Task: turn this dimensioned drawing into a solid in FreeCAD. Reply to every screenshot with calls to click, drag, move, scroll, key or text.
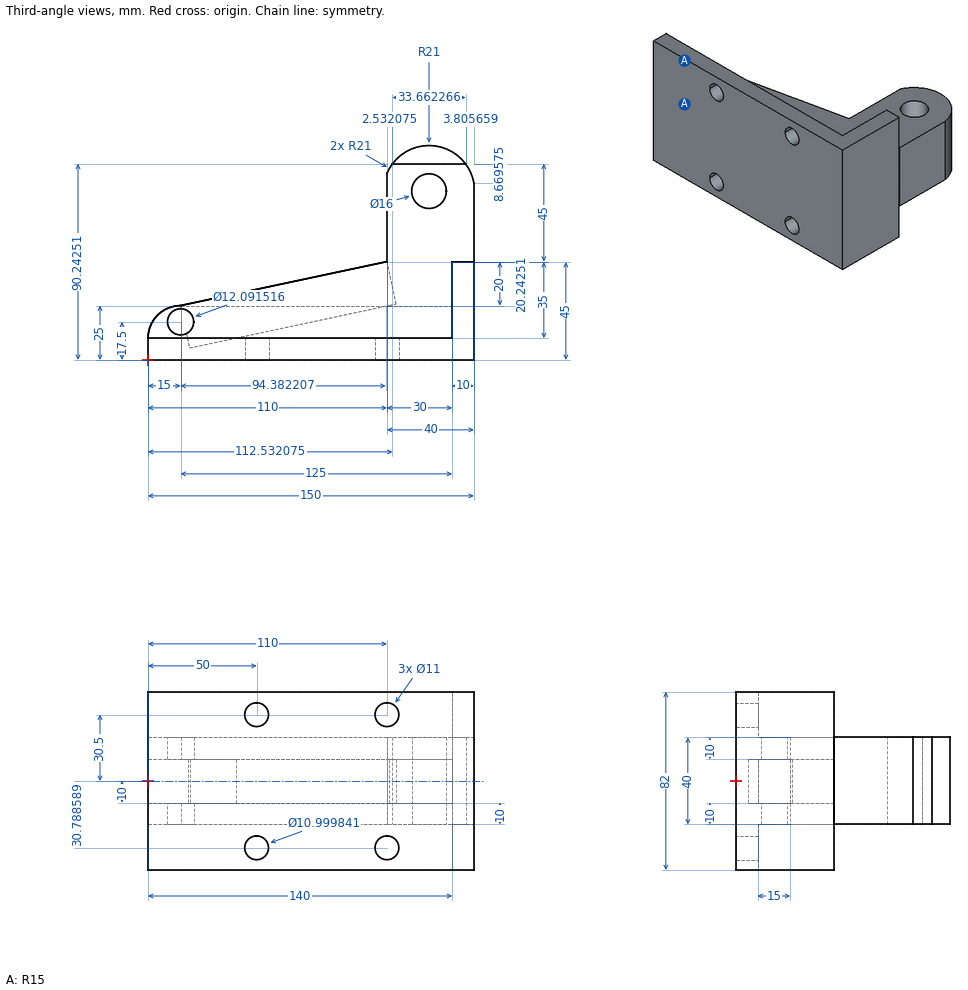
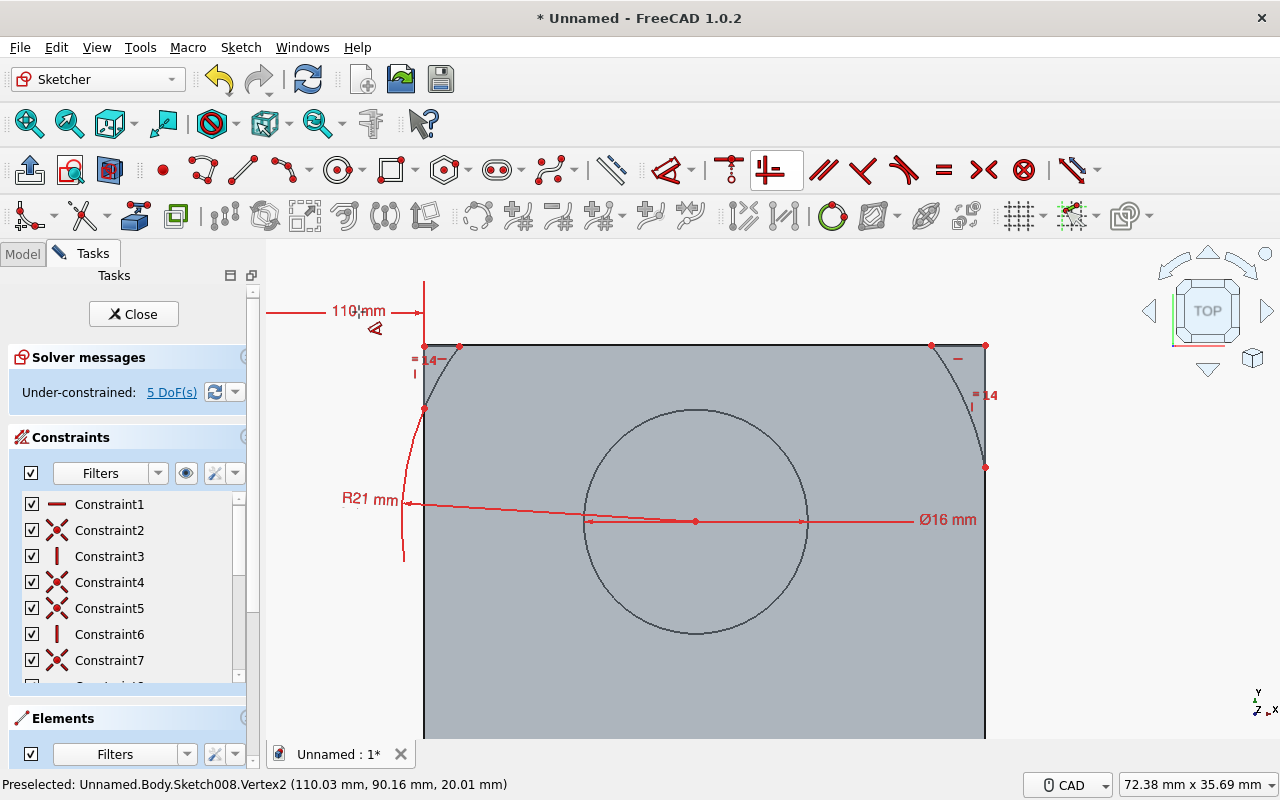
click(985, 468)
click(481, 434)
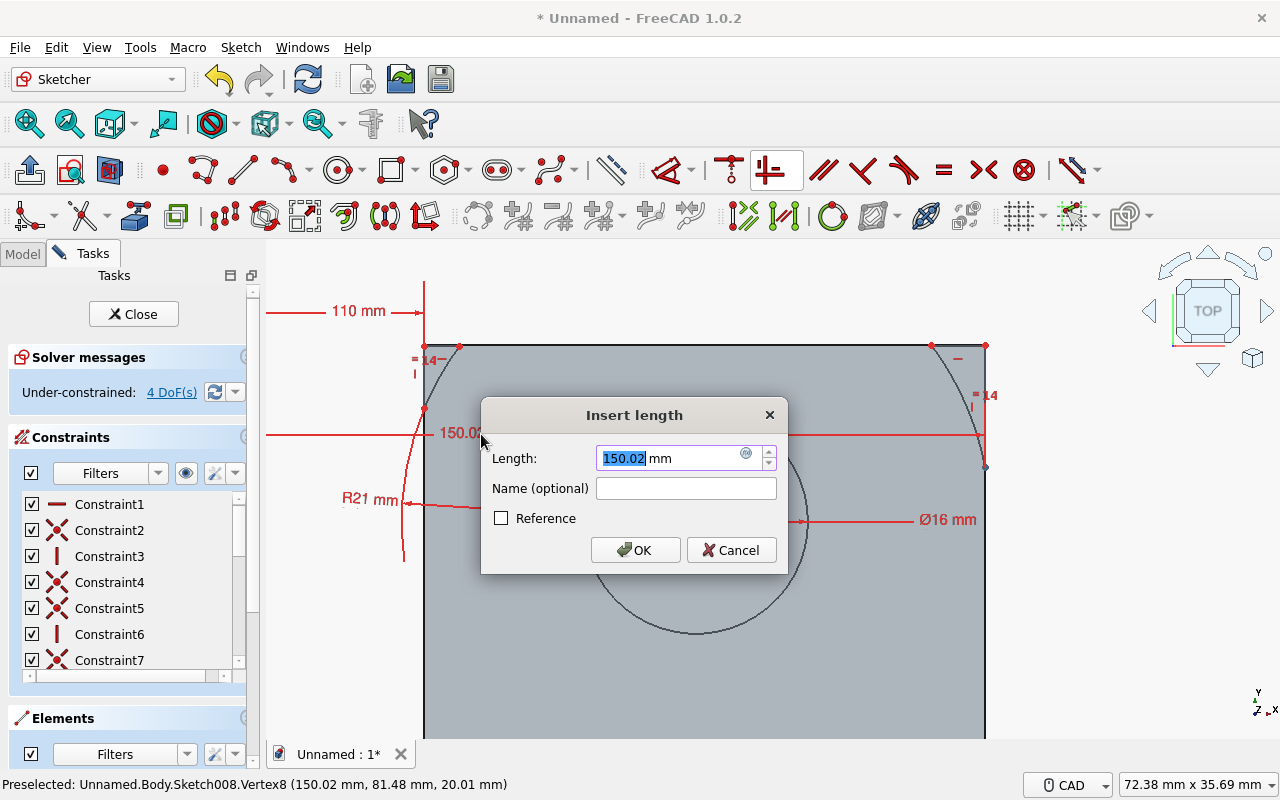
text(150)
key(Return)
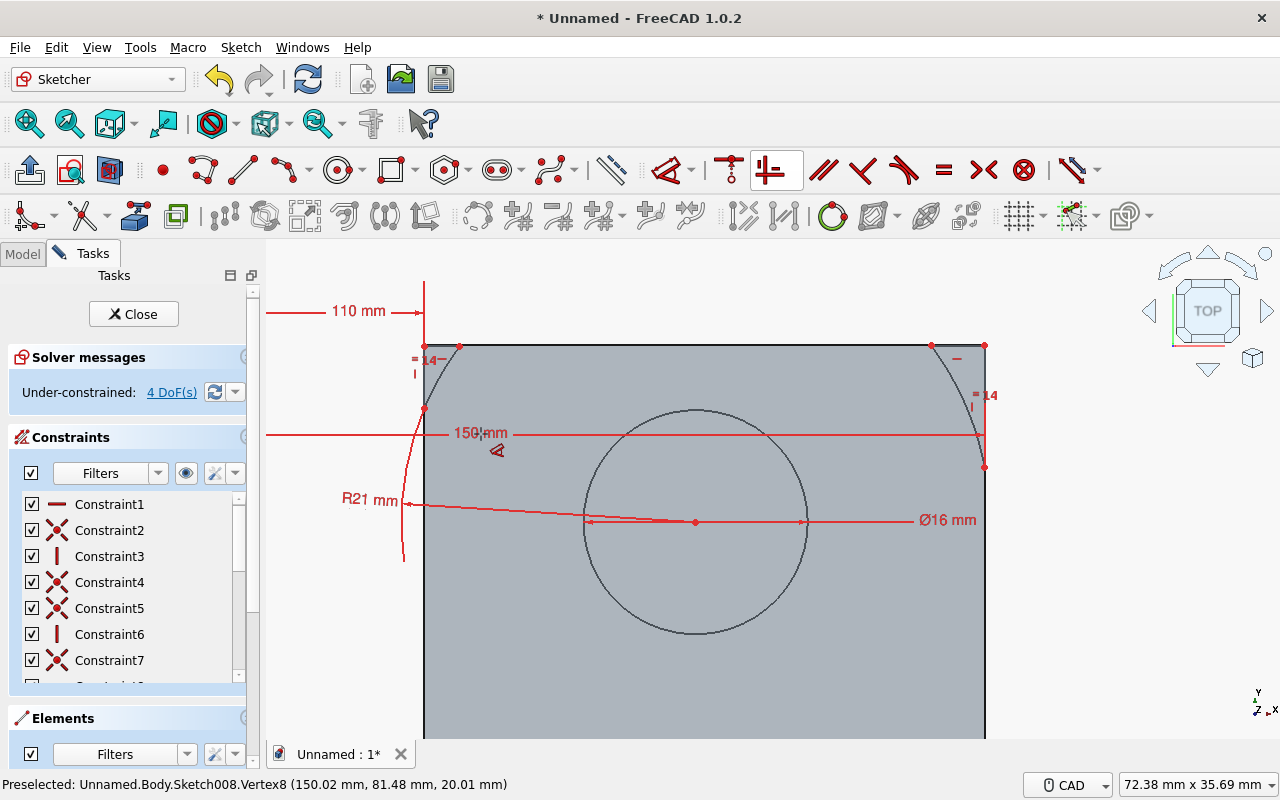
scroll(435, 346, up, 2)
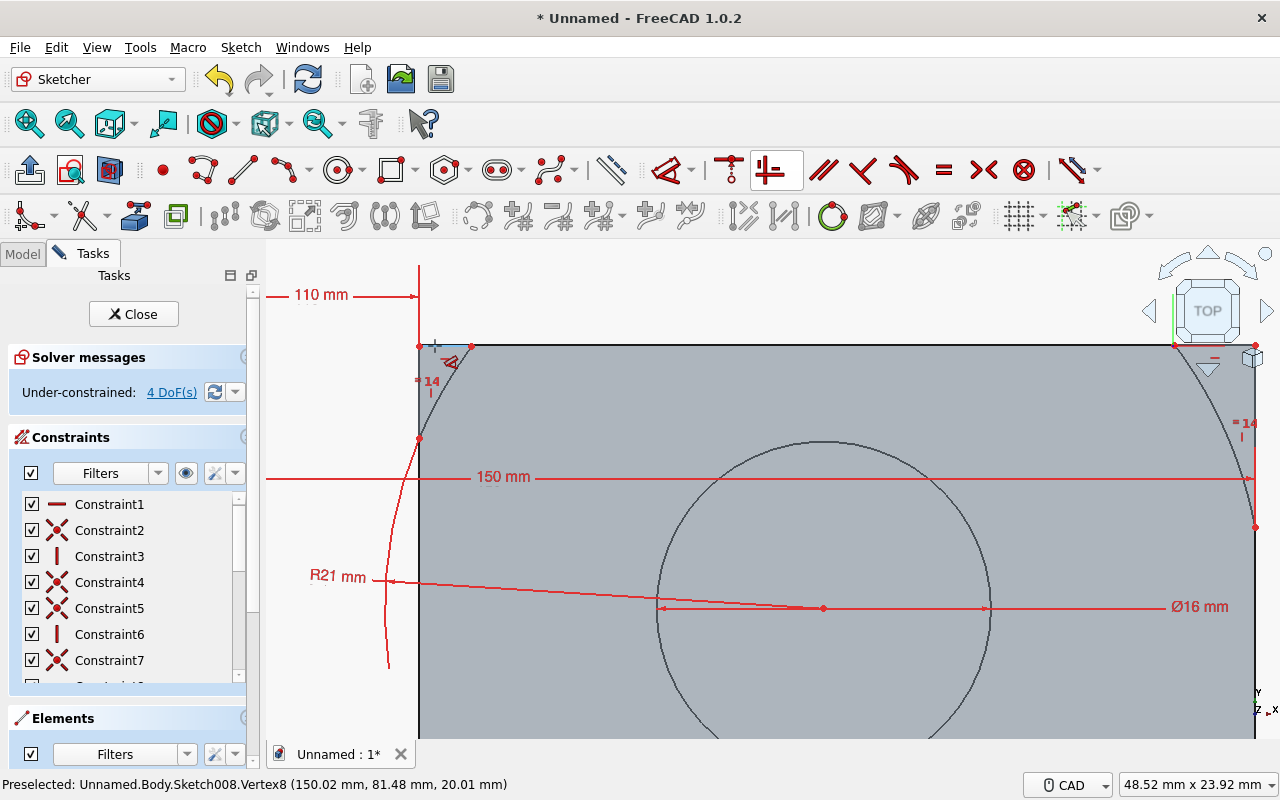
click(435, 346)
click(446, 312)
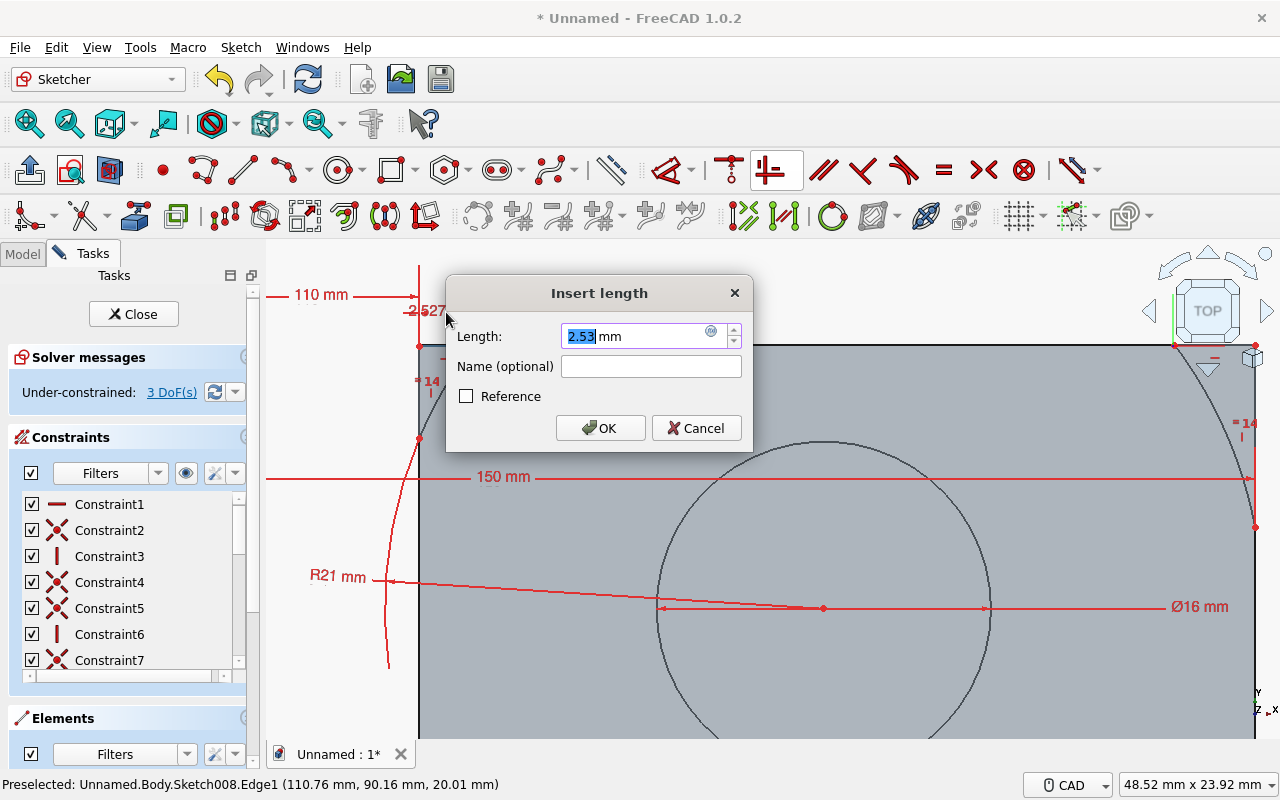
text(2.532075)
key(Return)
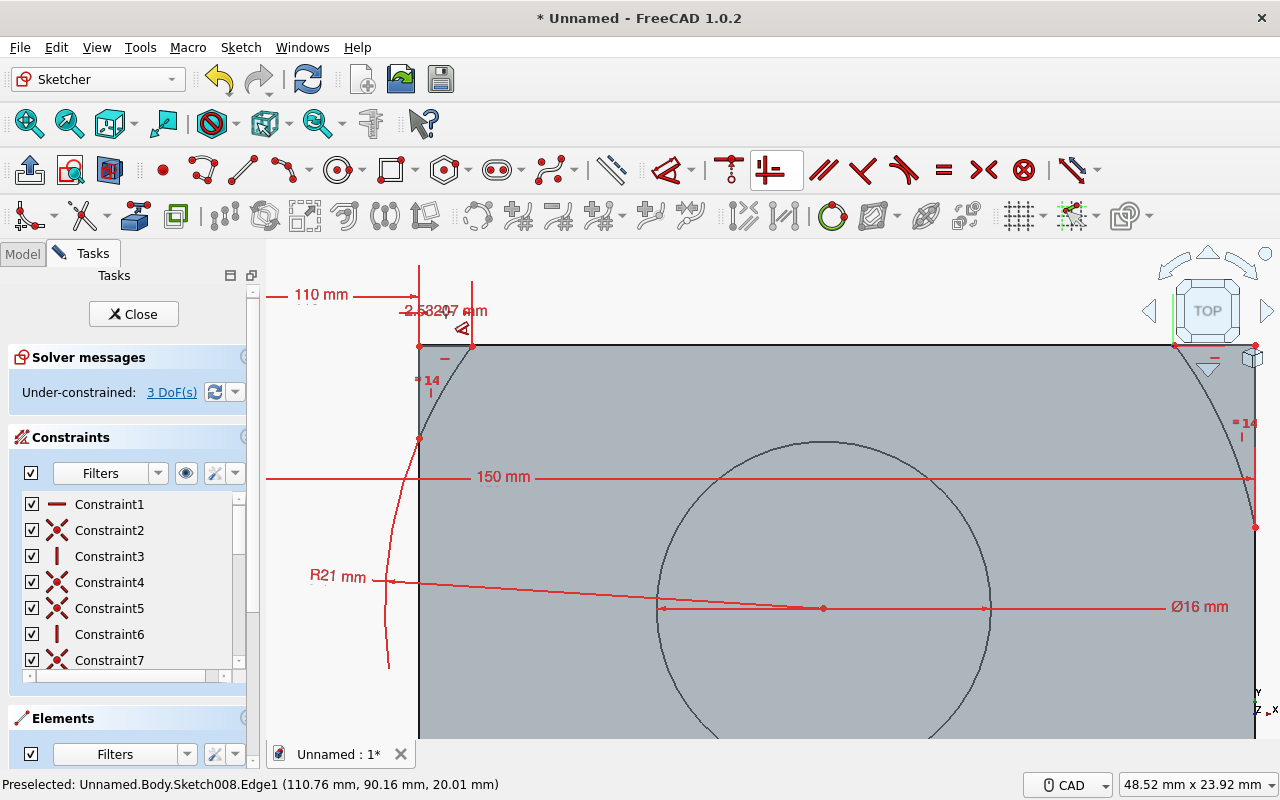
scroll(435, 346, down, 2)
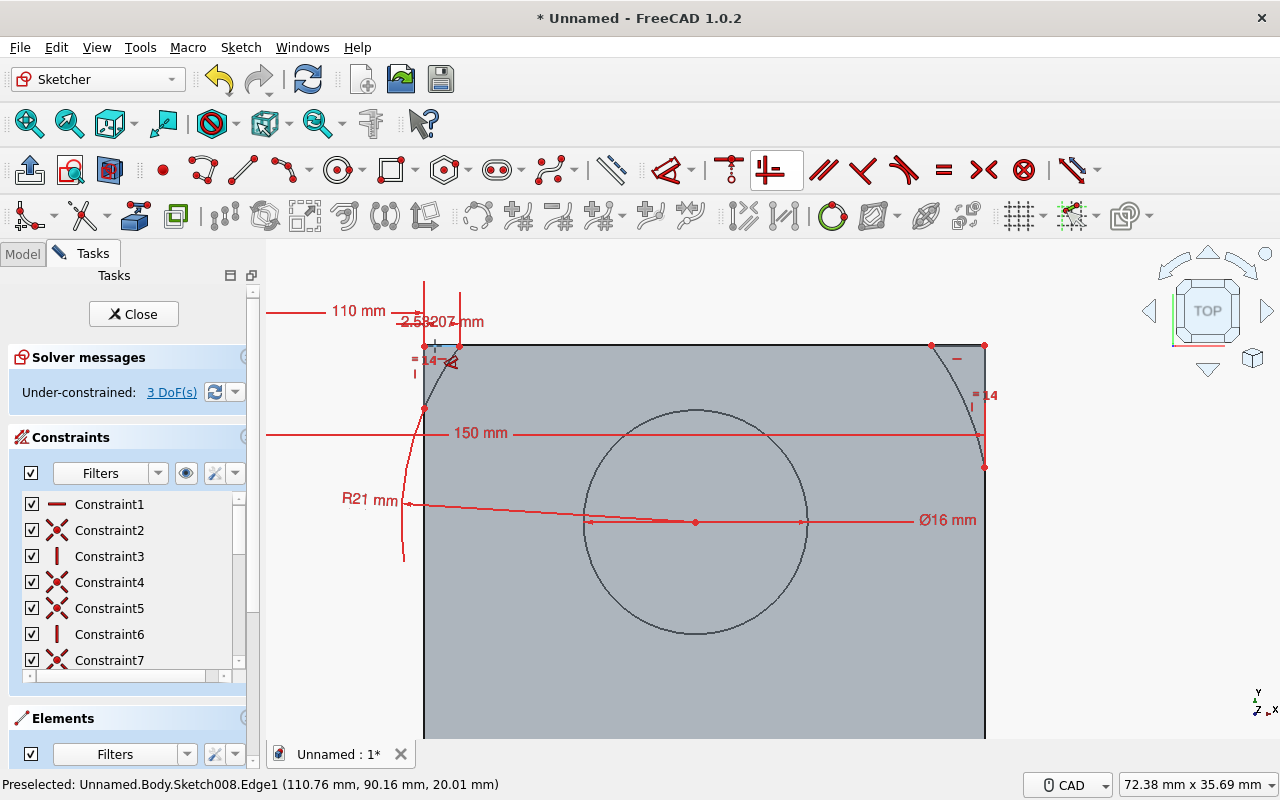
scroll(985, 431, up, 3)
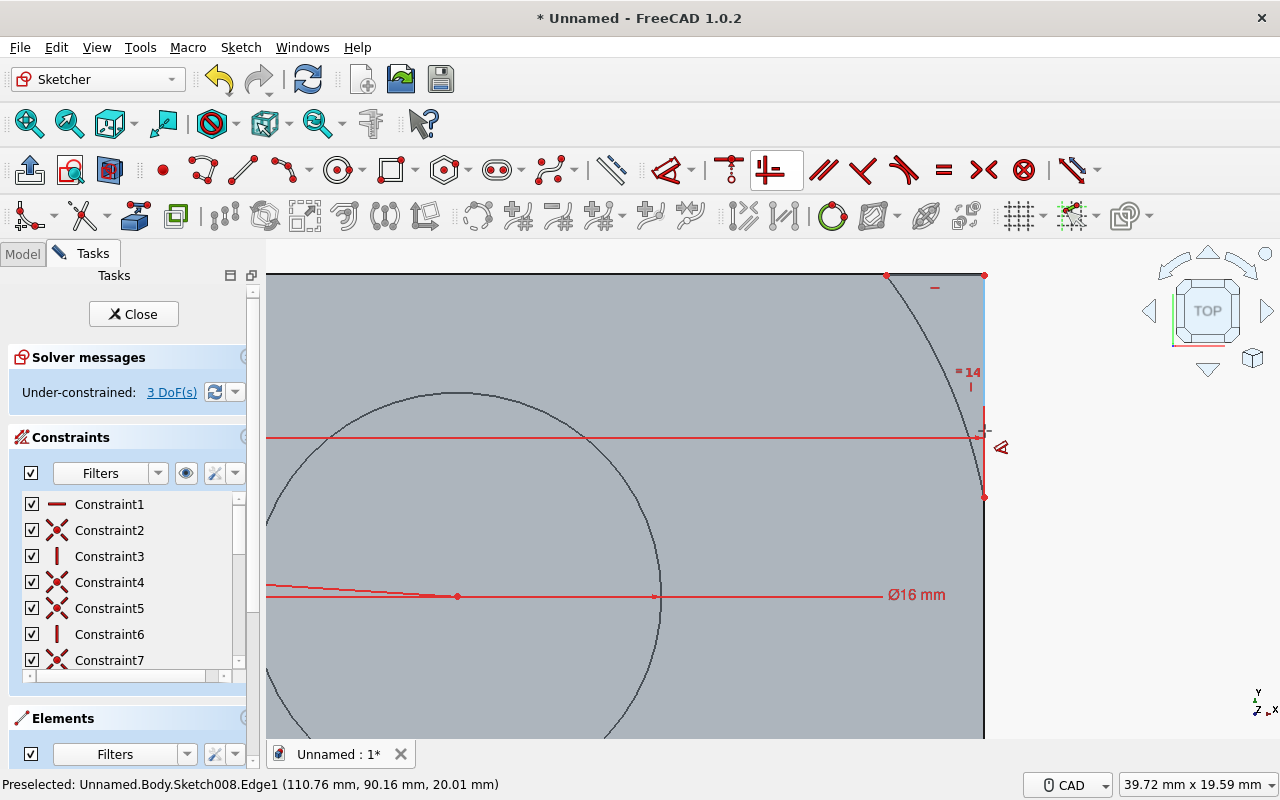
click(984, 431)
click(1018, 387)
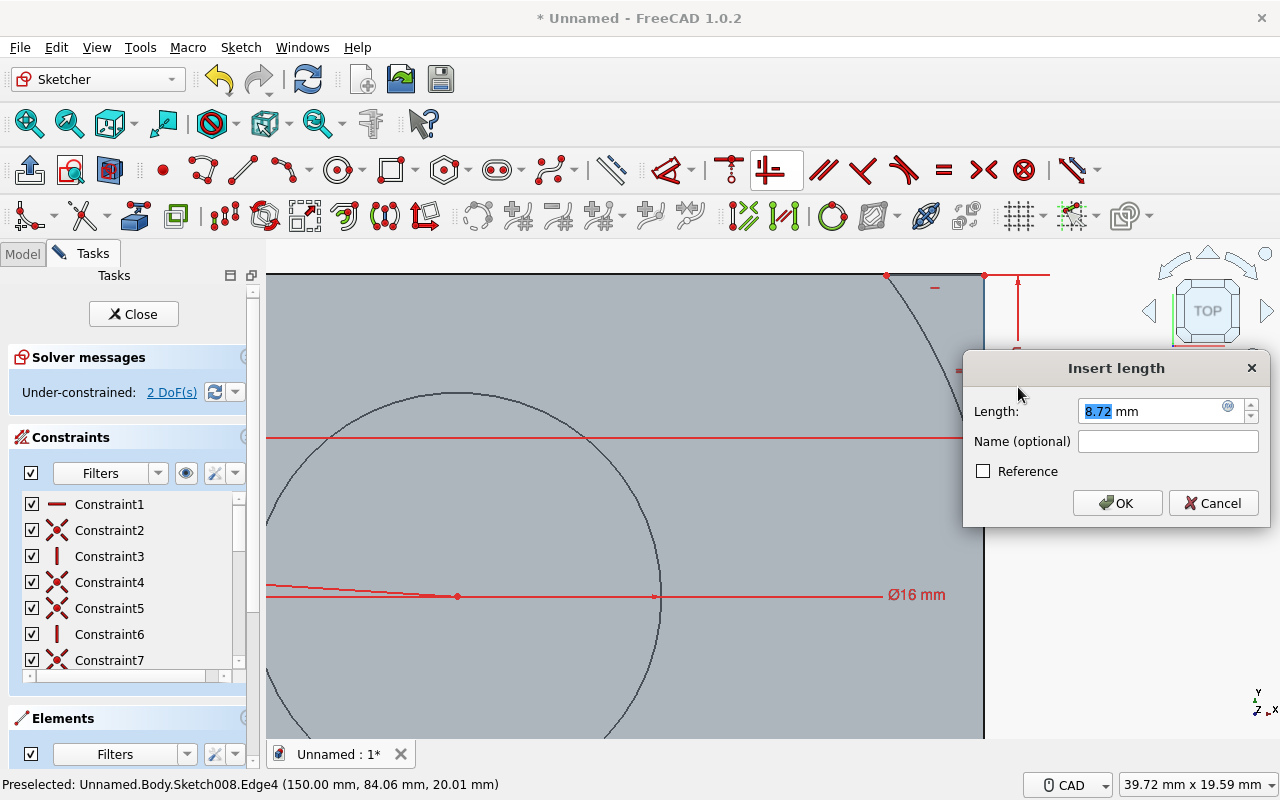
text(8.669575)
key(Return)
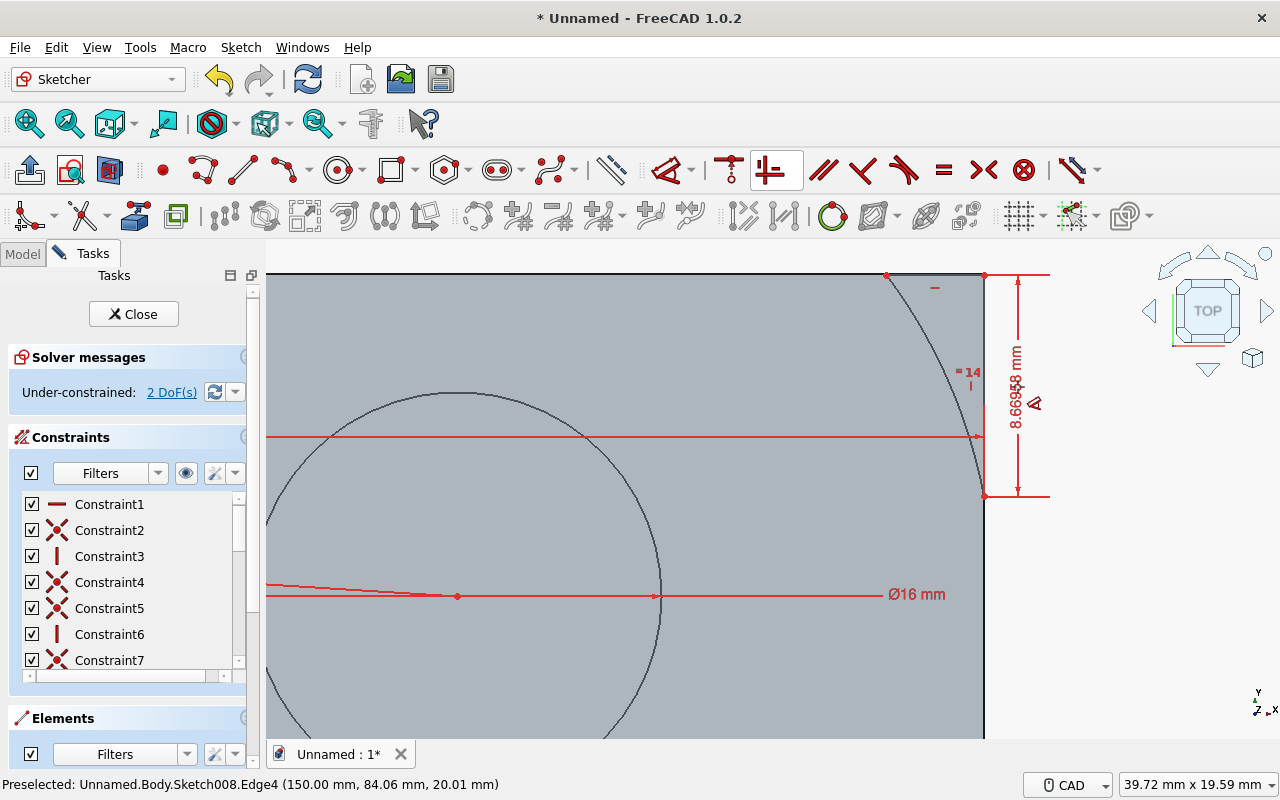
click(955, 275)
click(935, 309)